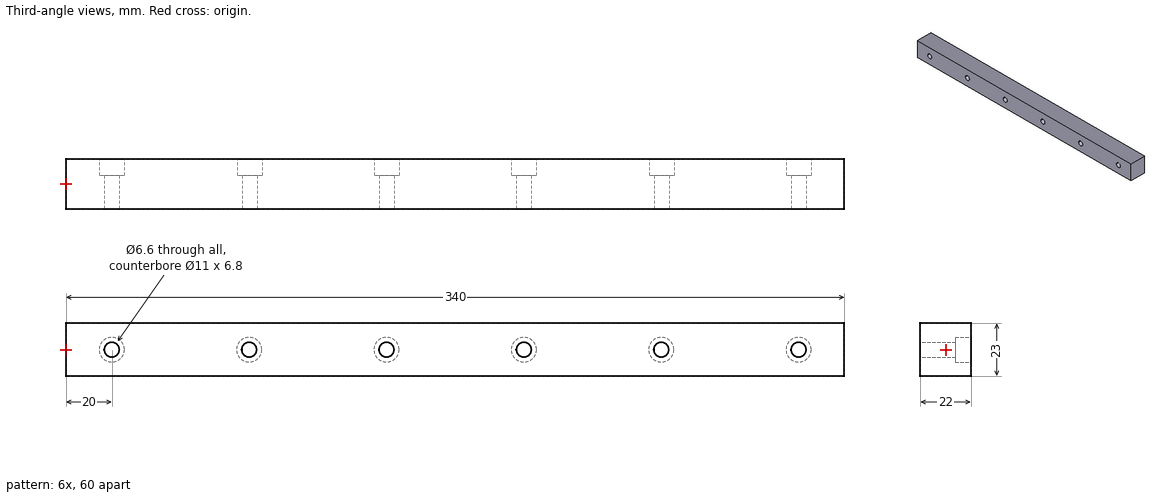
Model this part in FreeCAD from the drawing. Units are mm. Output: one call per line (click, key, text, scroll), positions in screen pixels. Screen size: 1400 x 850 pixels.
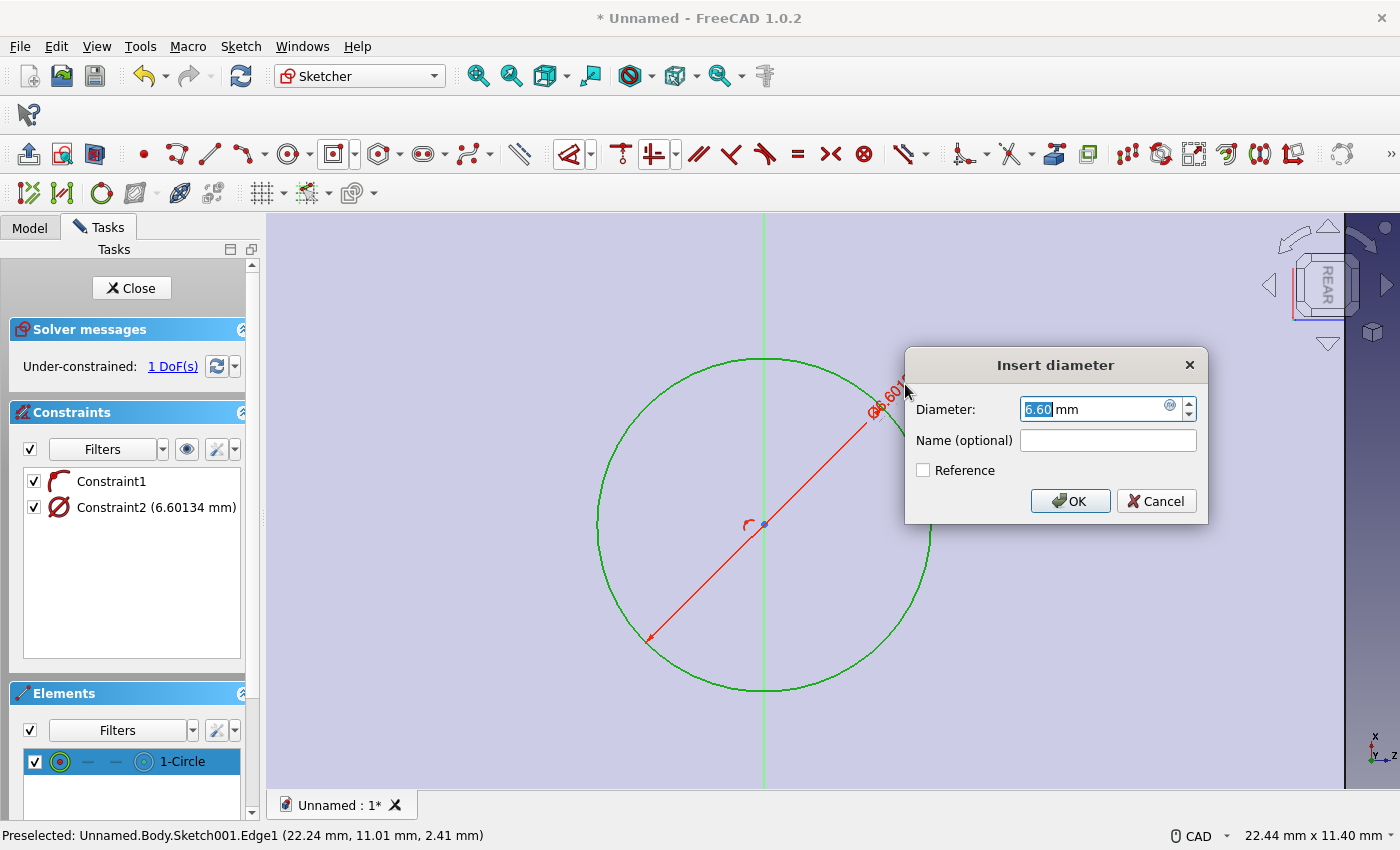
text(6.6)
key(Return)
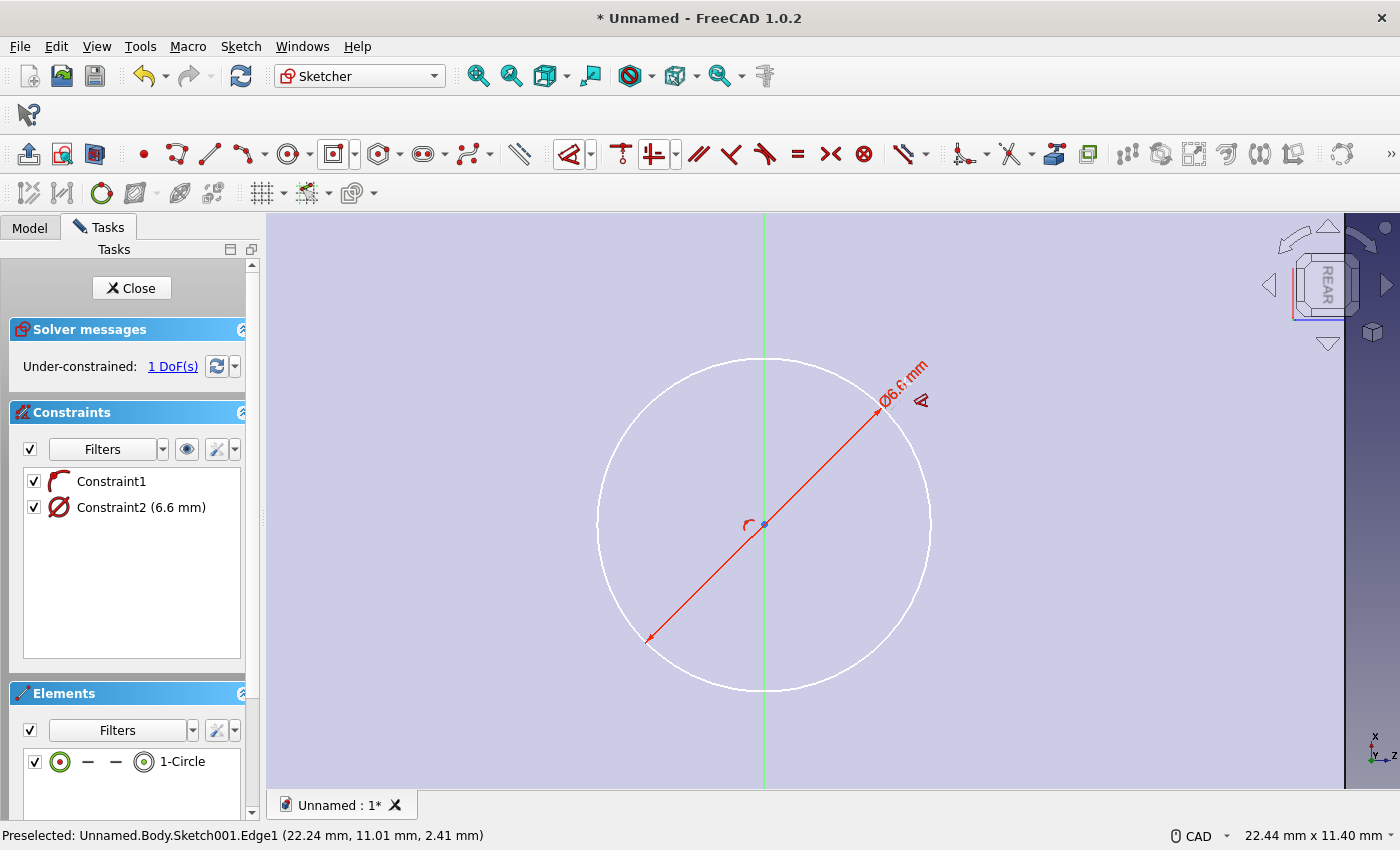
click(764, 525)
click(798, 643)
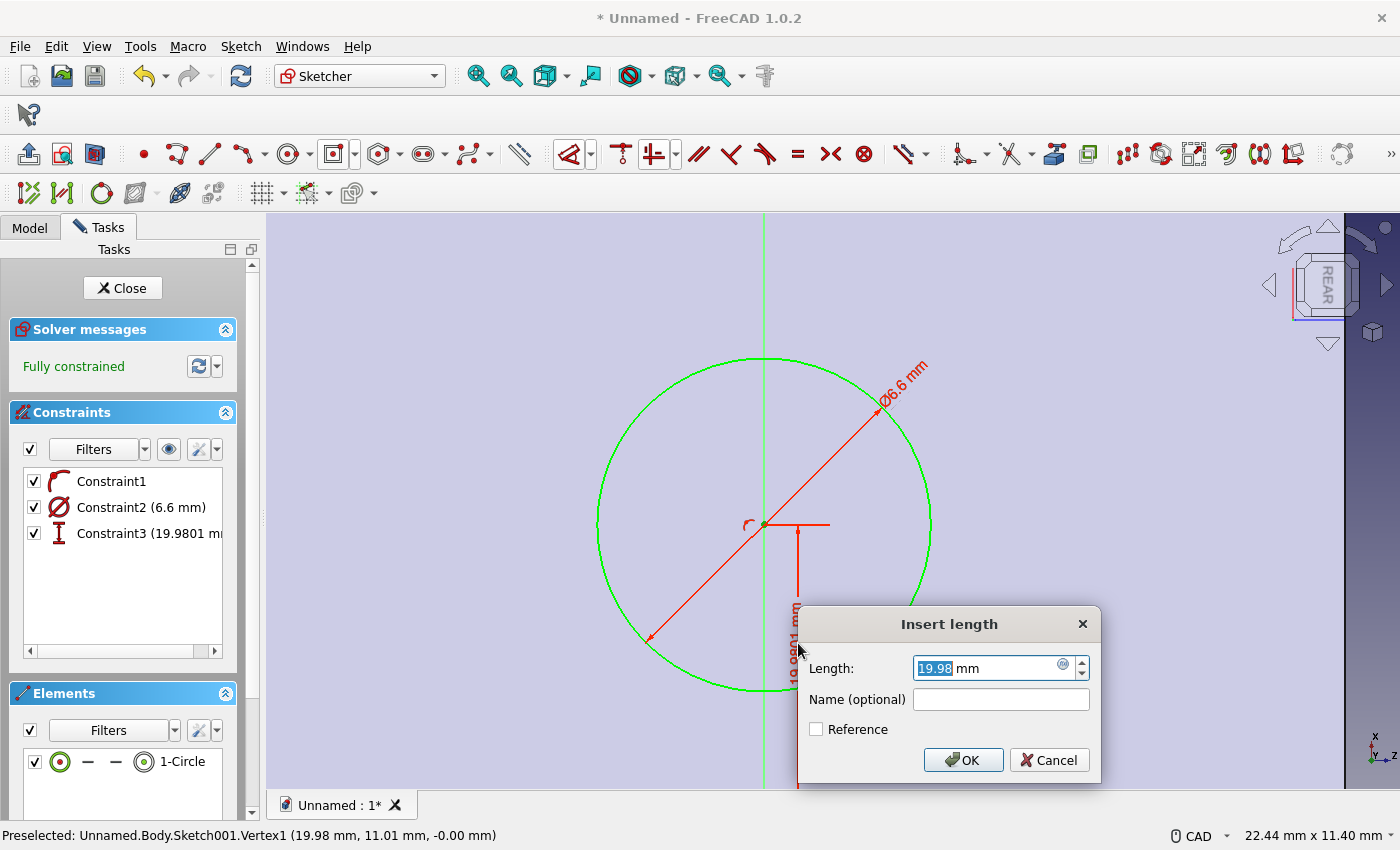
text(20)
key(Return)
key(Escape)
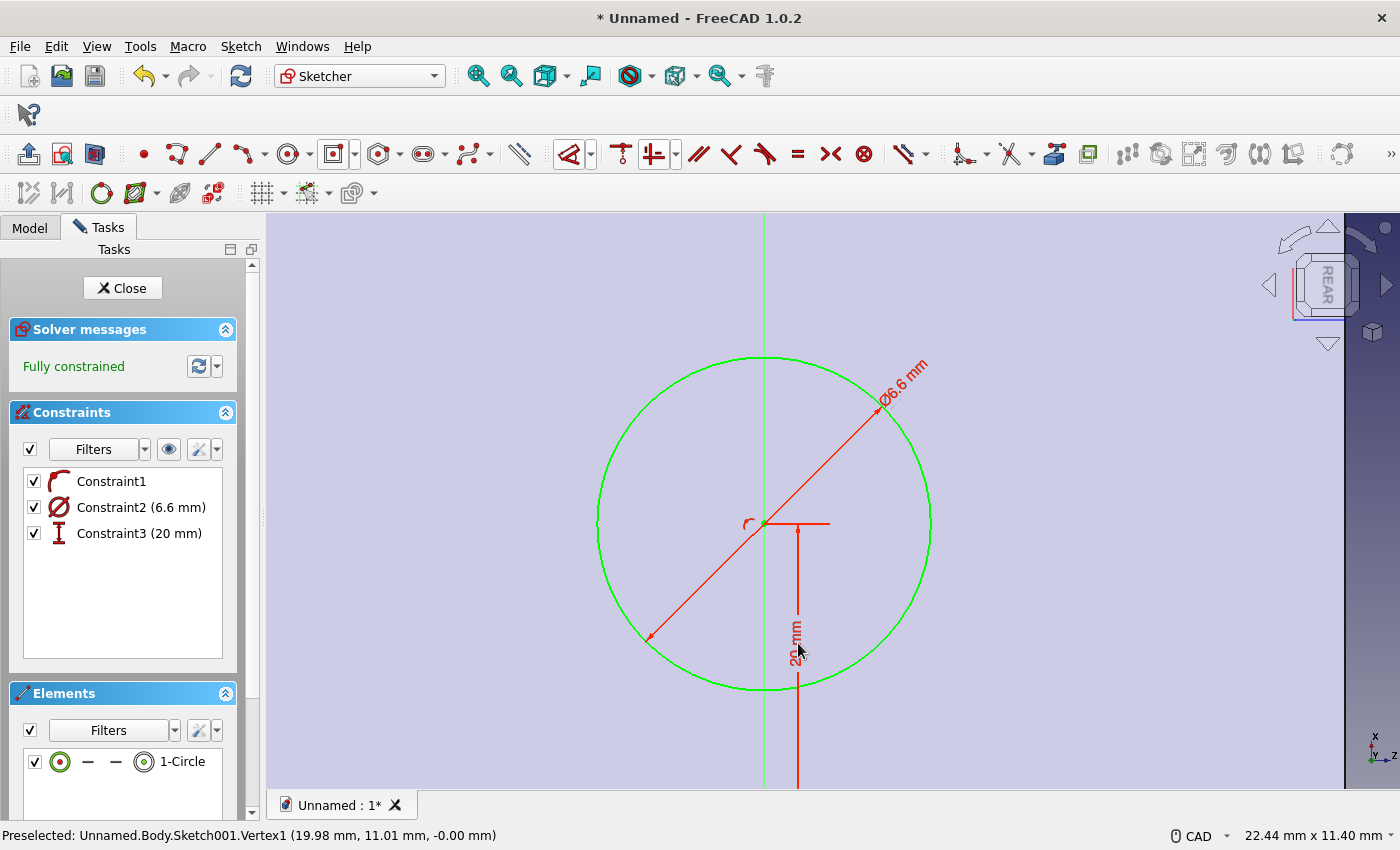
click(123, 288)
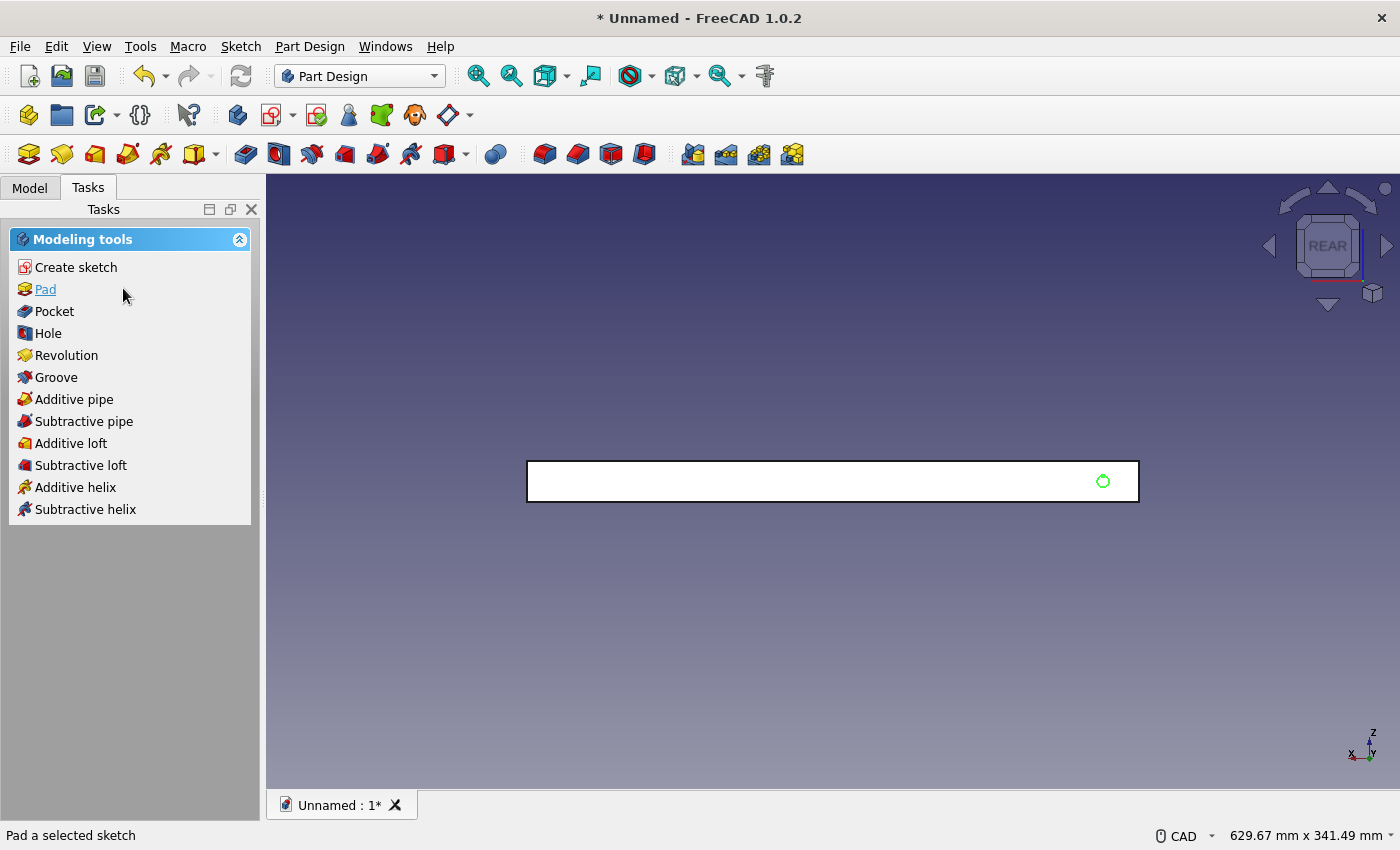
click(279, 154)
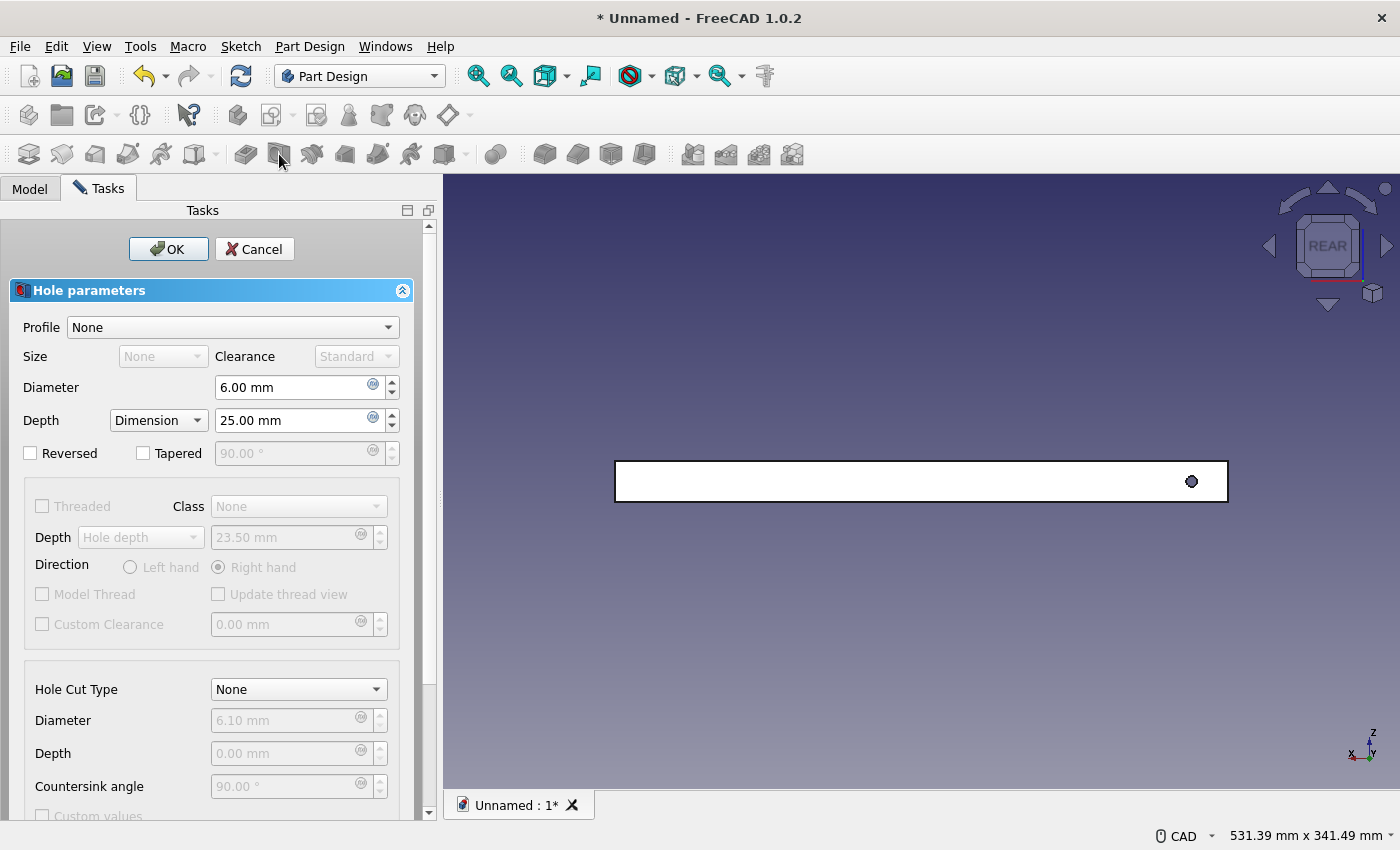
triple_click(300, 388)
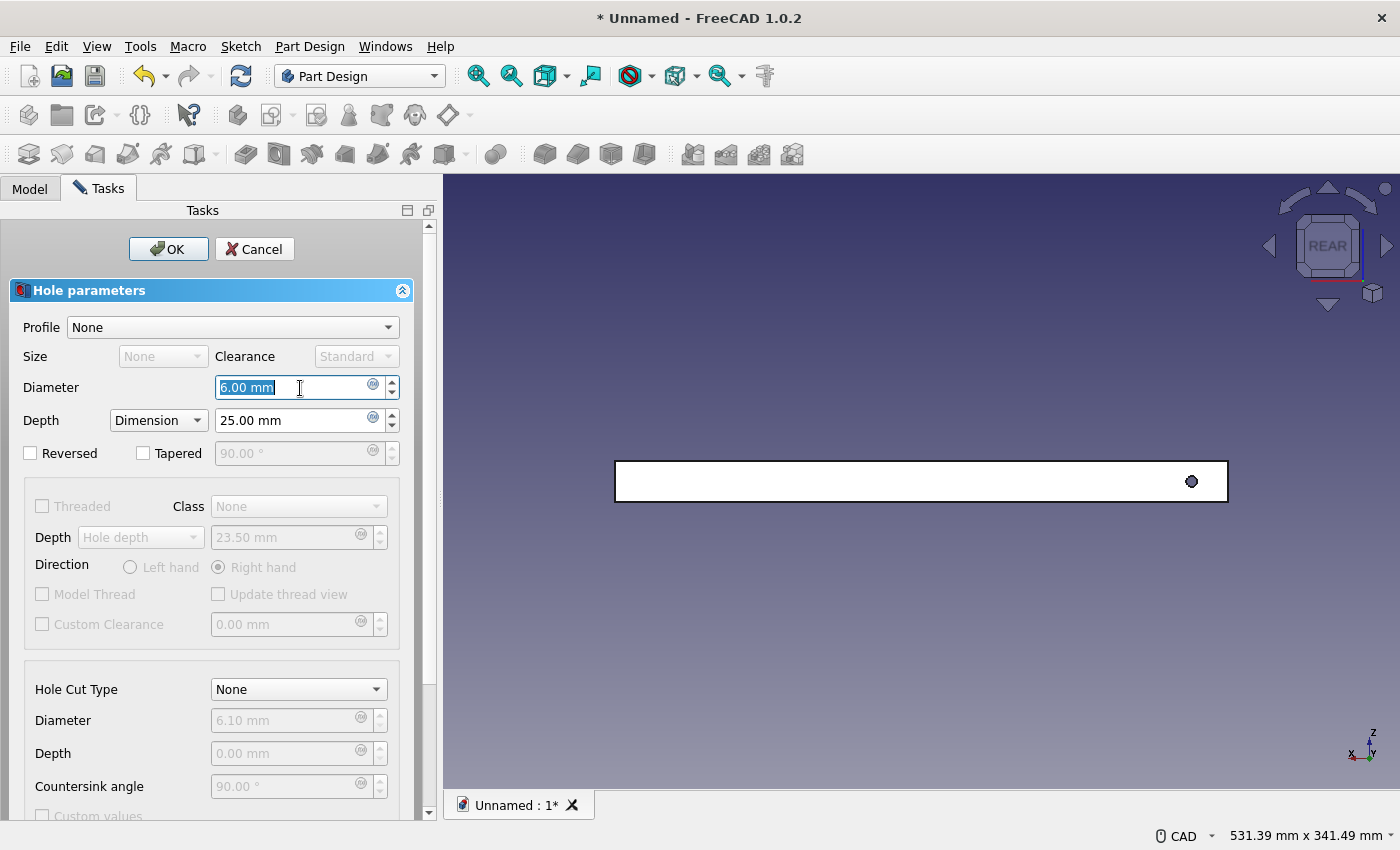
text(6.6)
key(Tab)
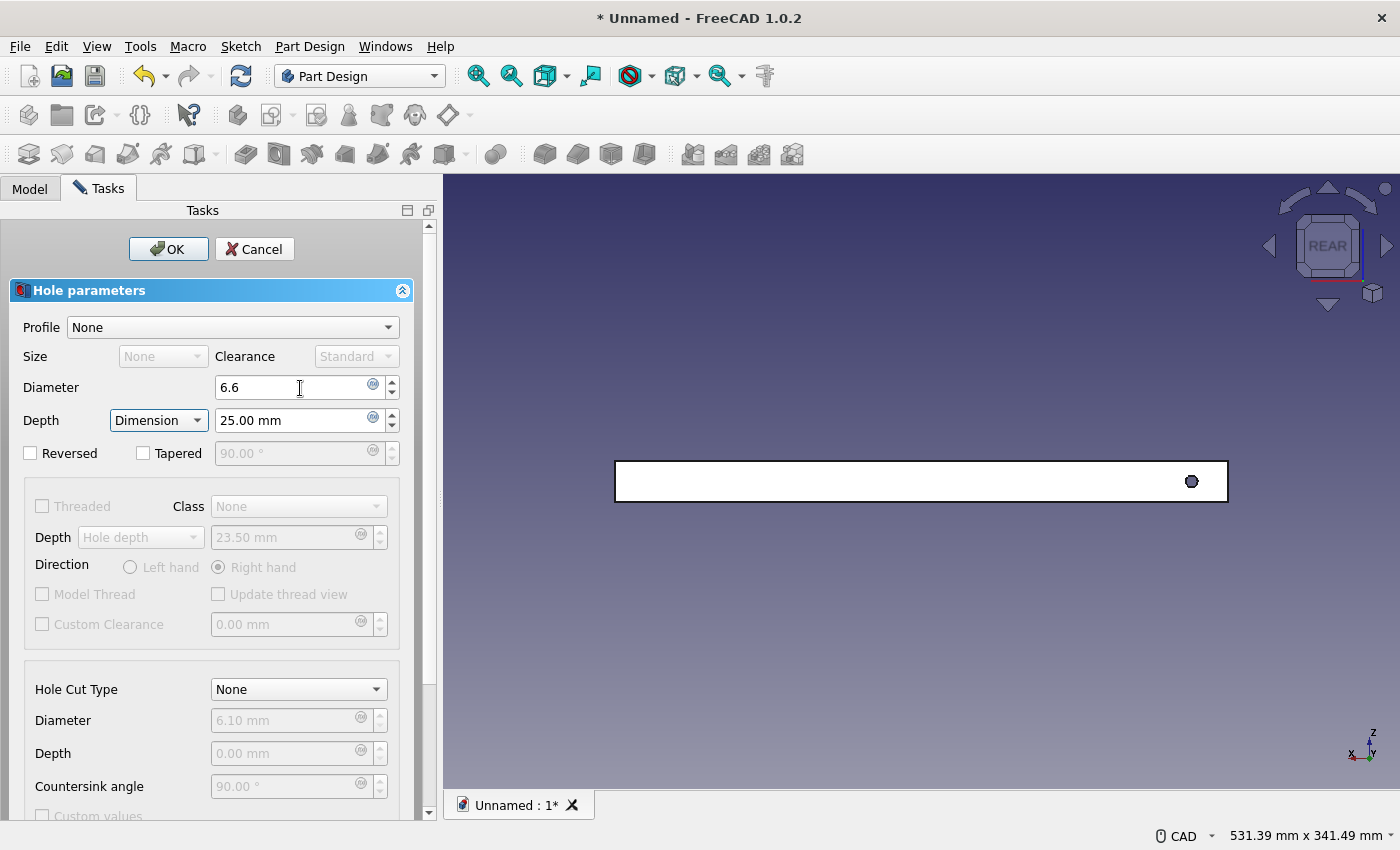
click(160, 420)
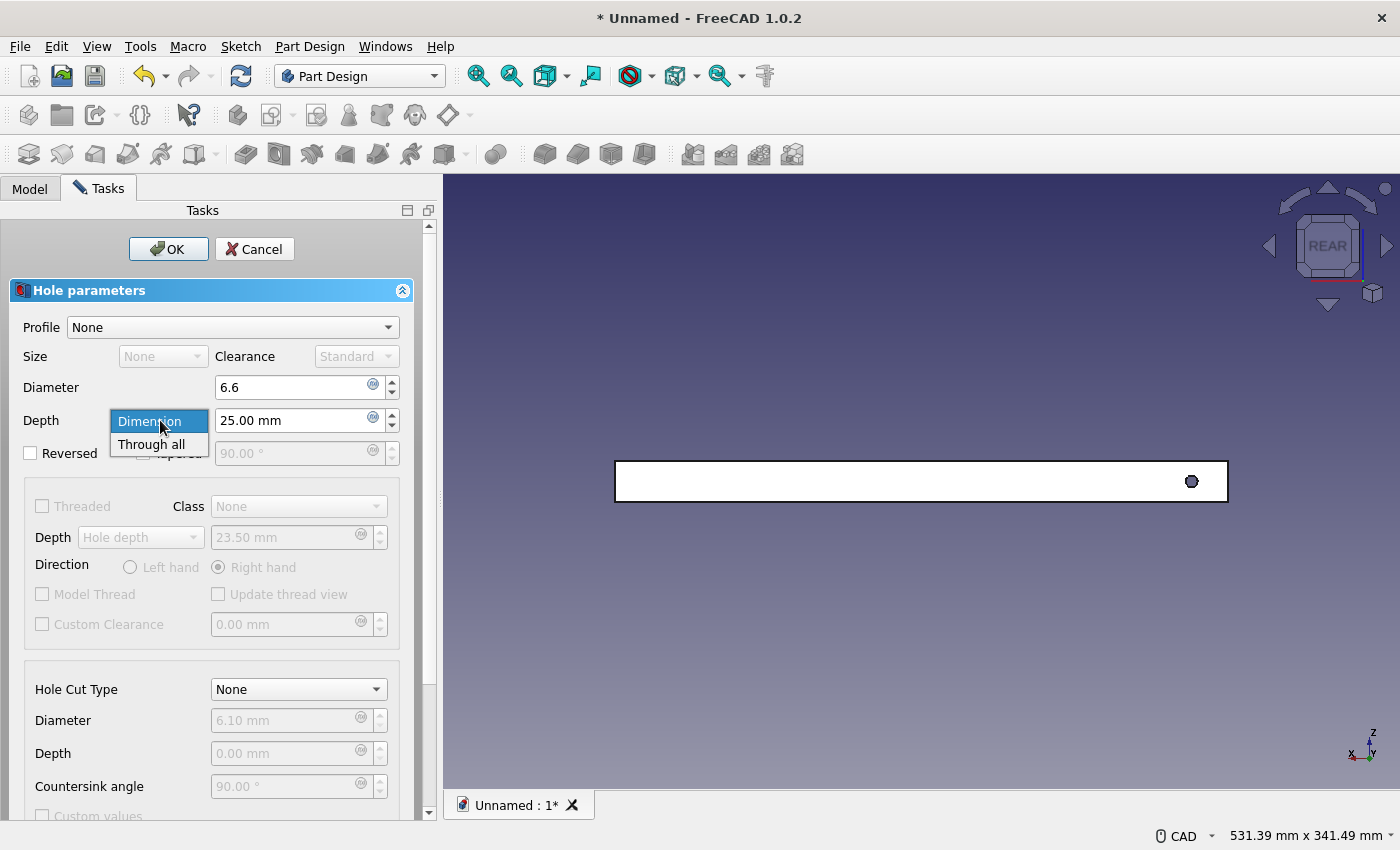
click(158, 444)